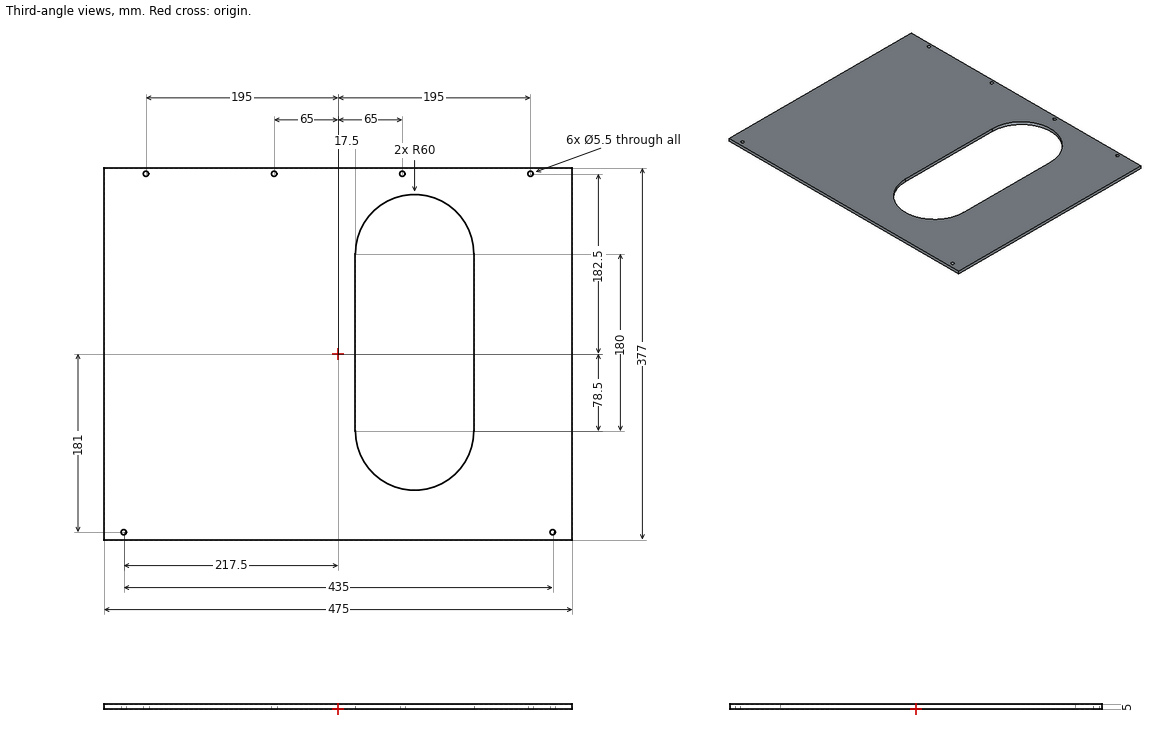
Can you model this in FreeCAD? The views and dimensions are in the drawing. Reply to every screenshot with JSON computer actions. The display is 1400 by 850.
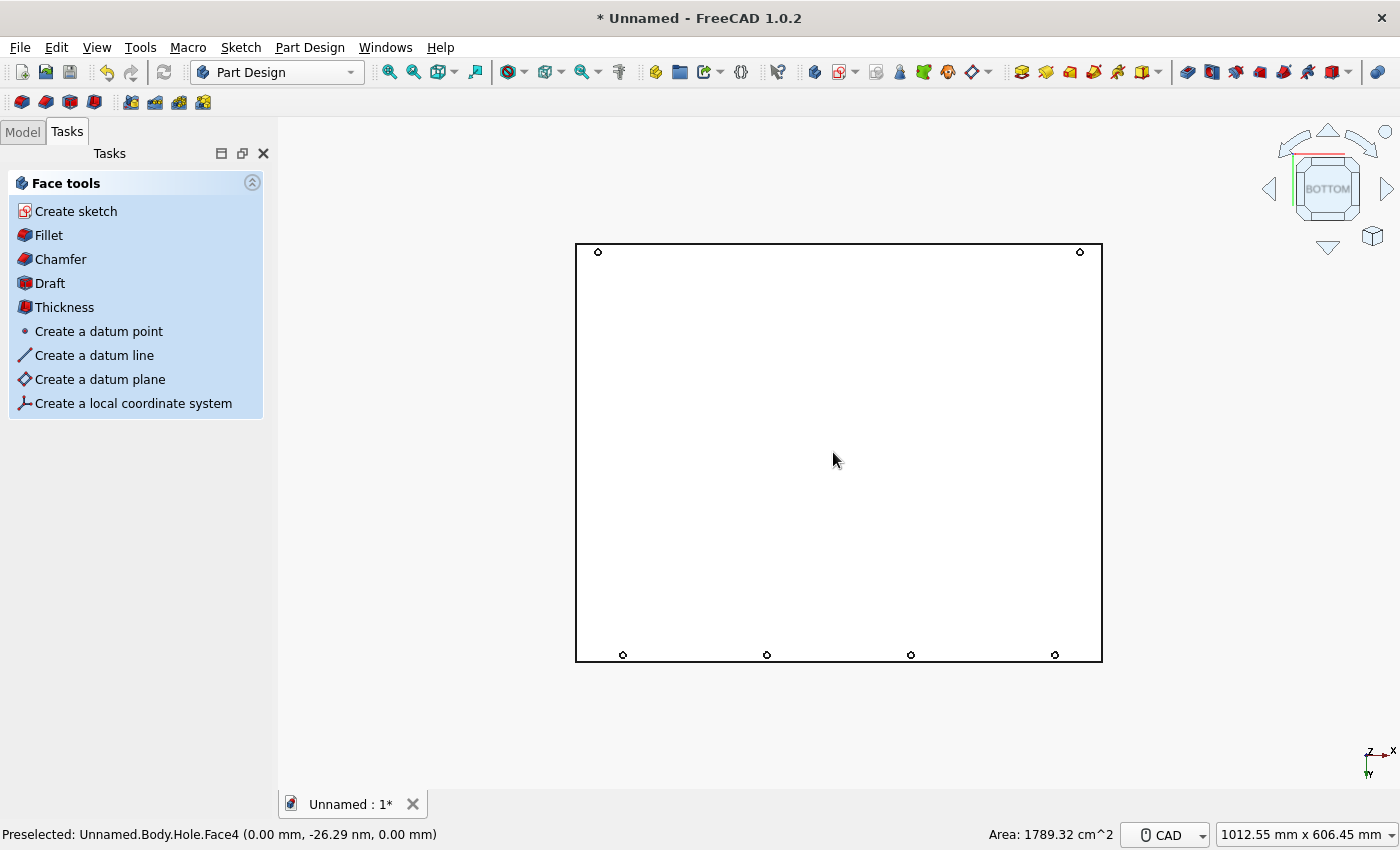
{"action": "left_click", "coordinate": [840, 72]}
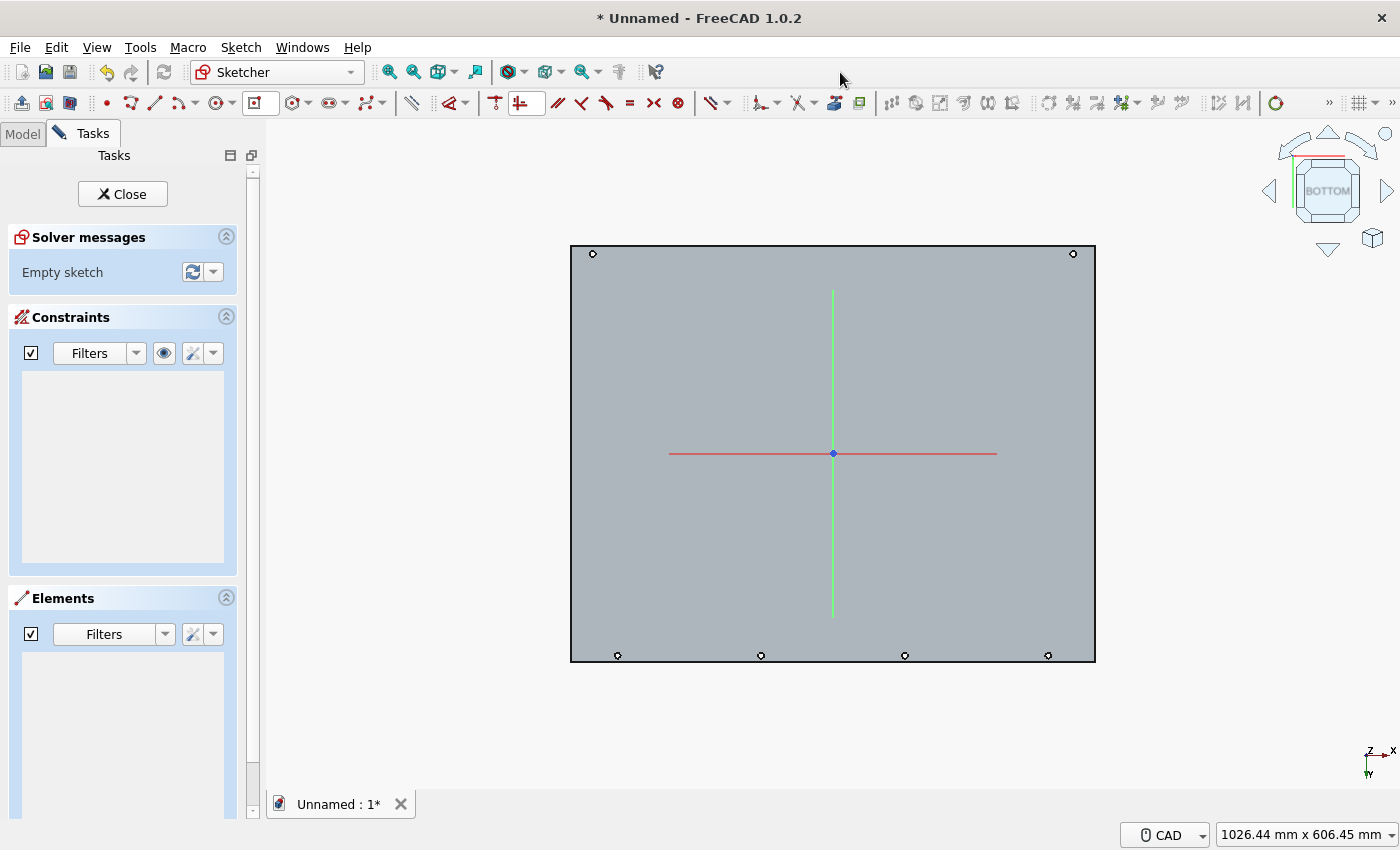
{"action": "left_click", "coordinate": [330, 104]}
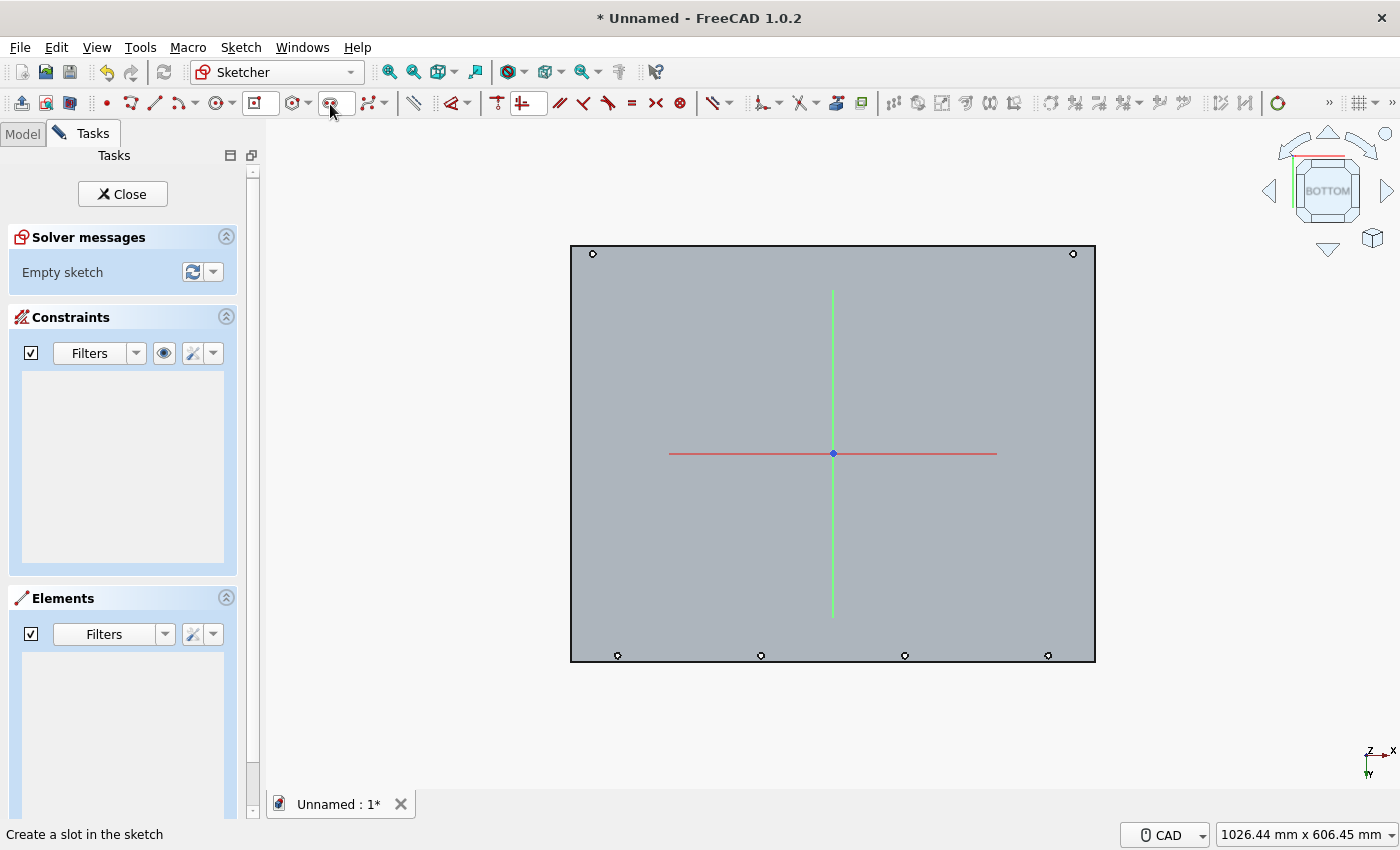
{"action": "left_click", "coordinate": [919, 566]}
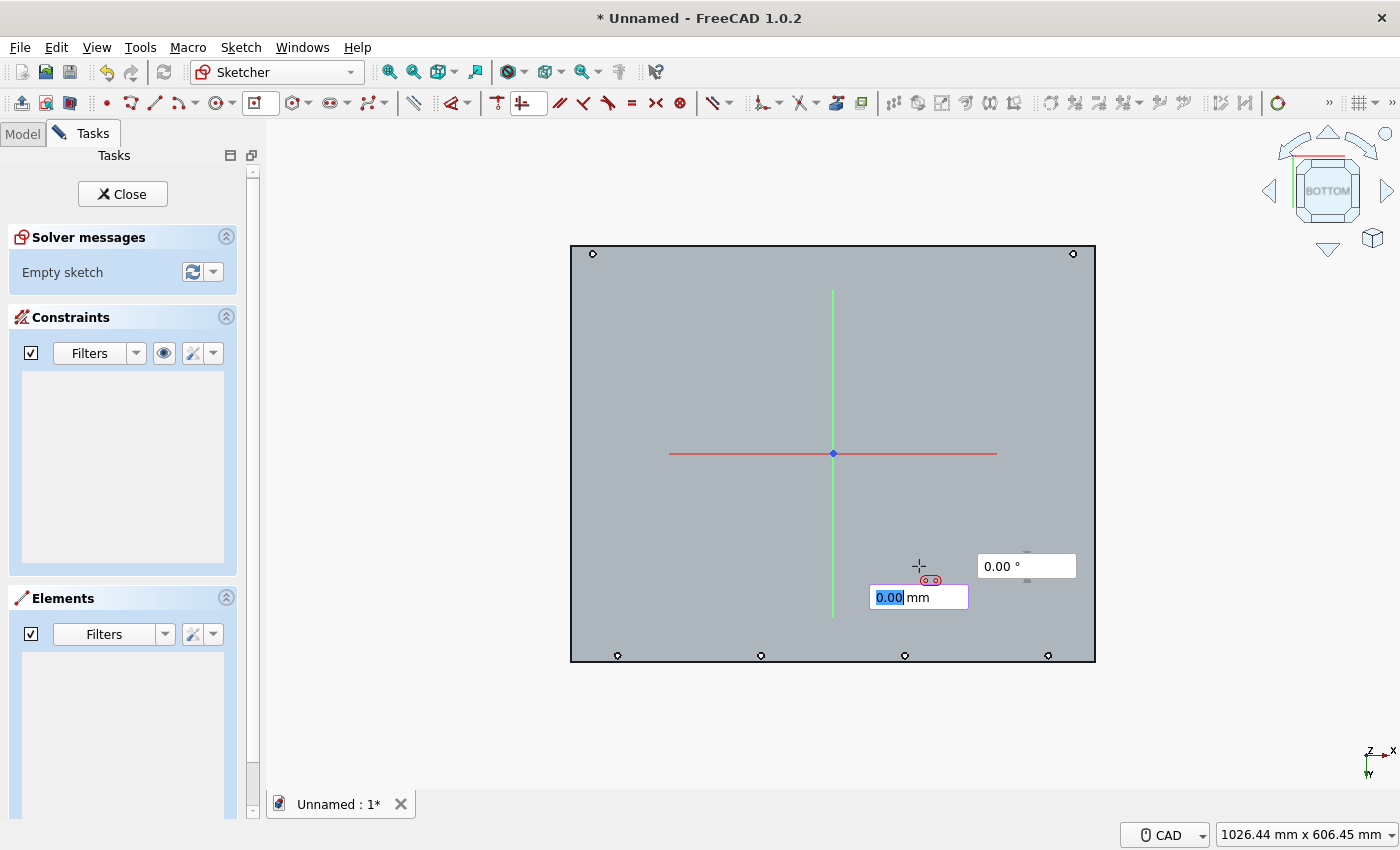
{"action": "left_click", "coordinate": [919, 367]}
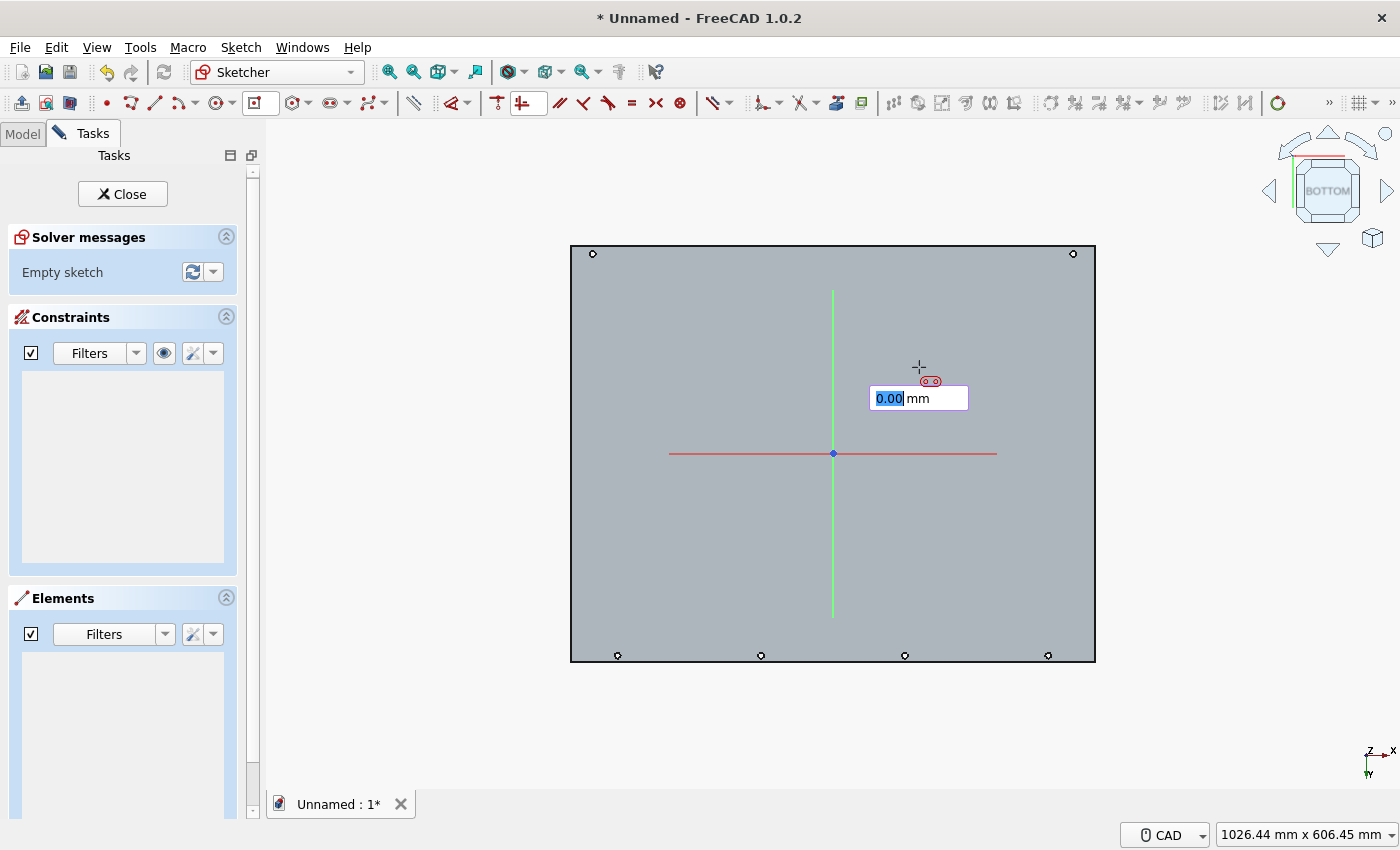
{"action": "left_click", "coordinate": [852, 437]}
{"action": "key", "text": "Escape"}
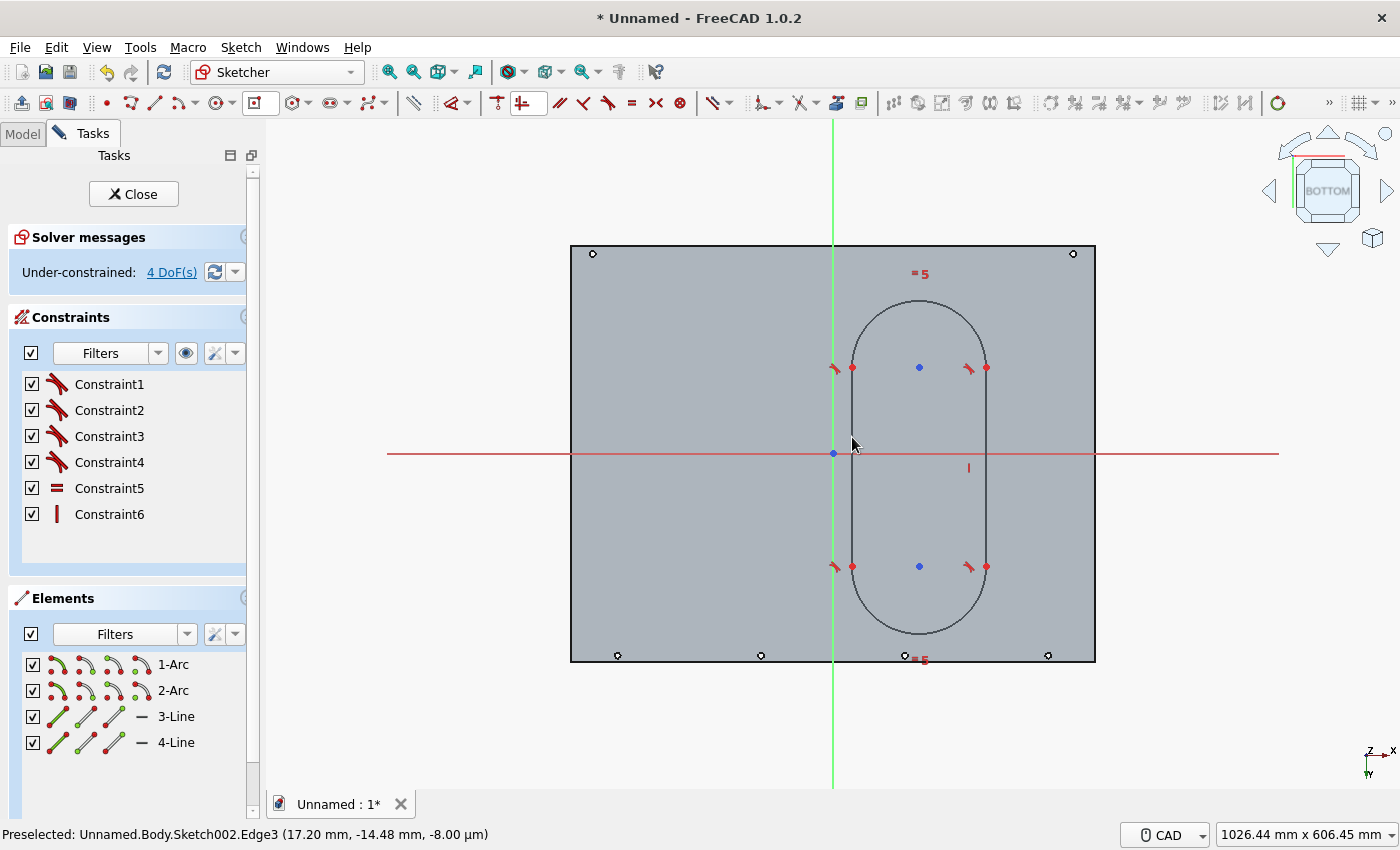
{"action": "left_click", "coordinate": [880, 621]}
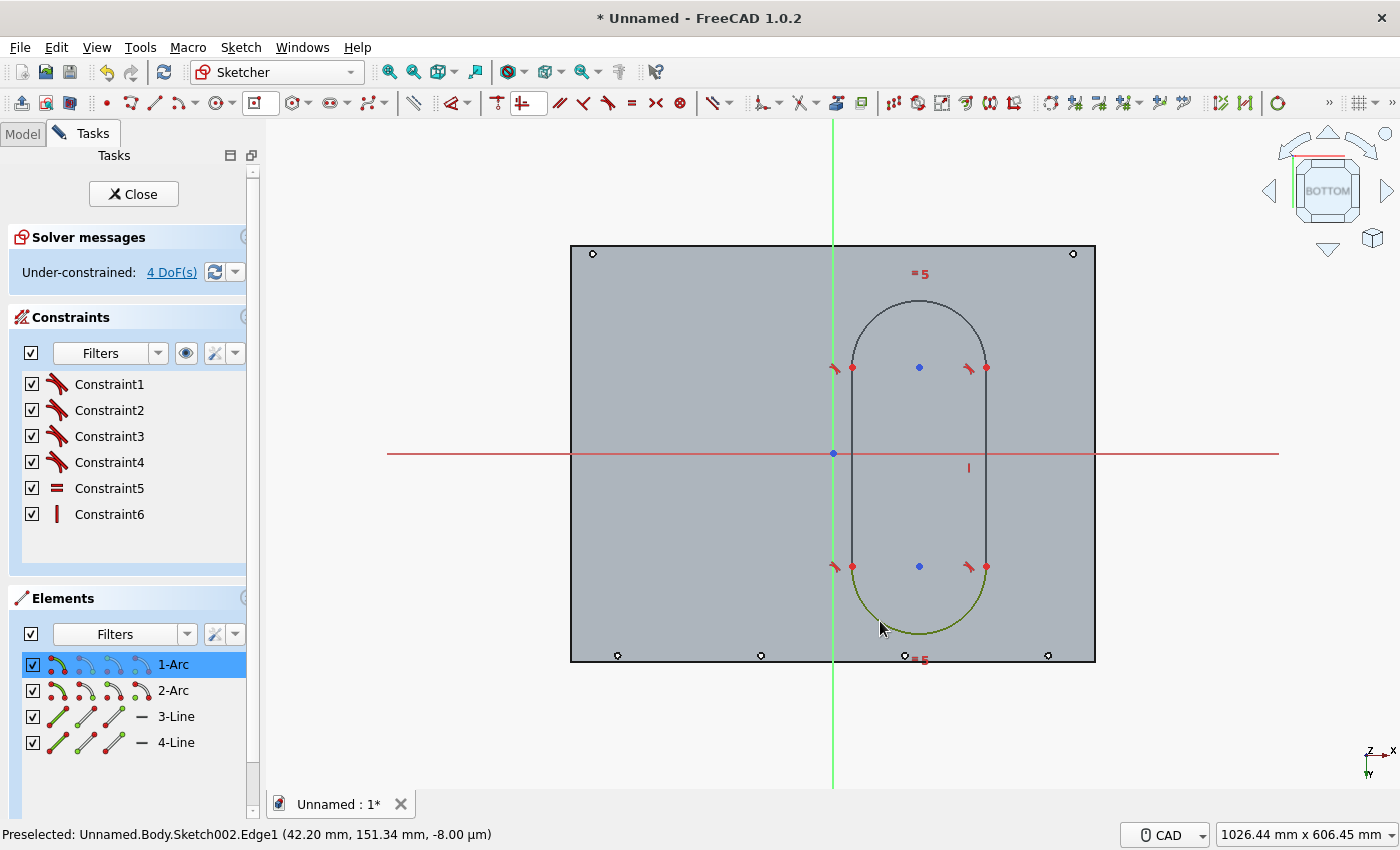
{"action": "key", "text": "k r"}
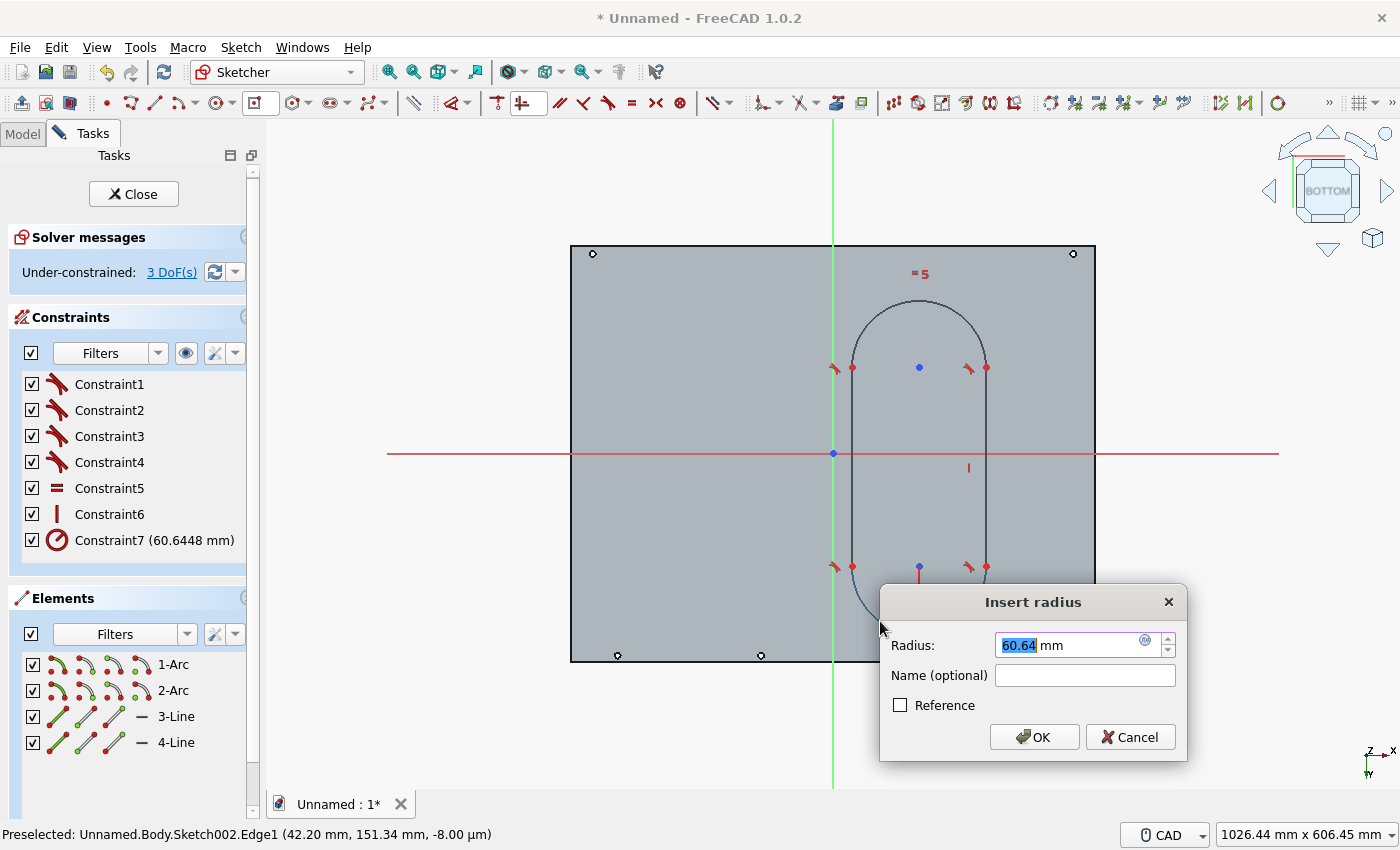
{"action": "type", "text": "60"}
{"action": "key", "text": "Return"}